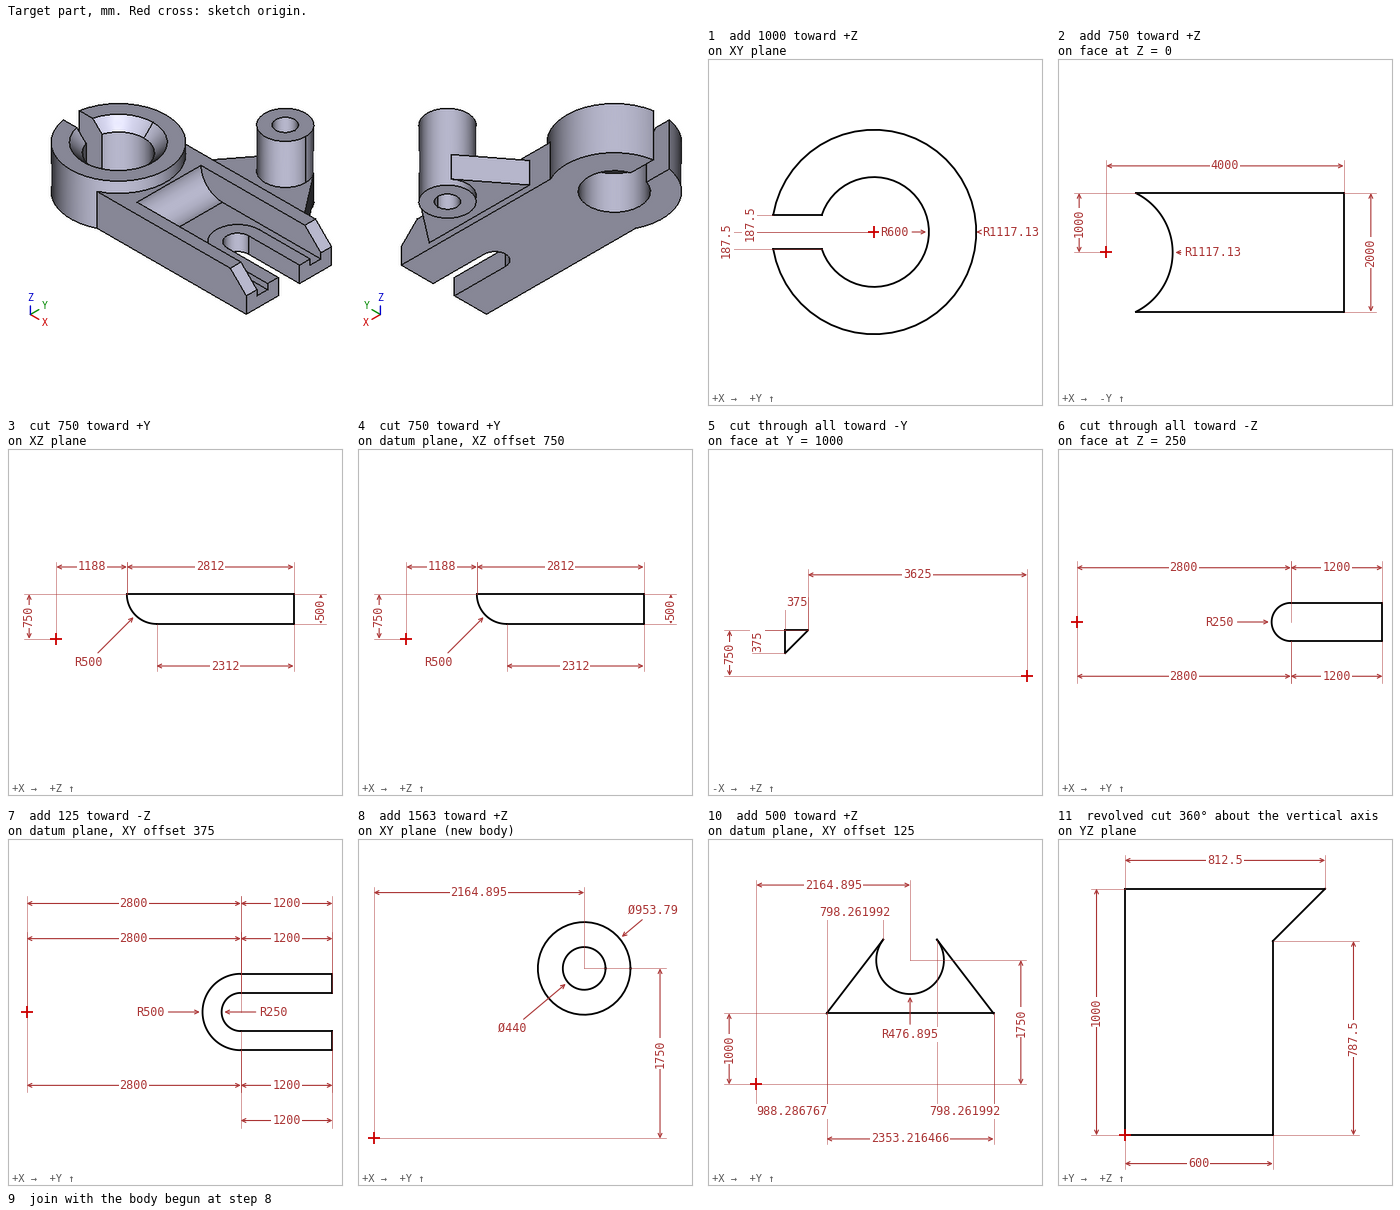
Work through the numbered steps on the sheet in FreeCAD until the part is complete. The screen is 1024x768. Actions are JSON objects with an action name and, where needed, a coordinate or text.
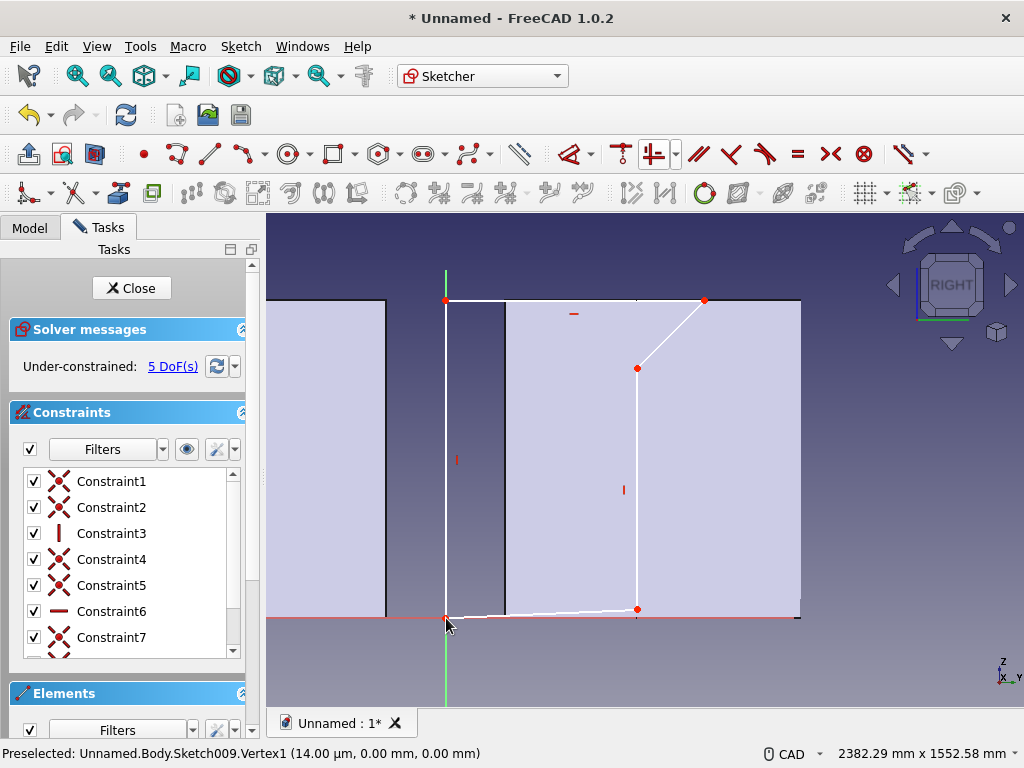
{"action": "left_click", "coordinate": [503, 616]}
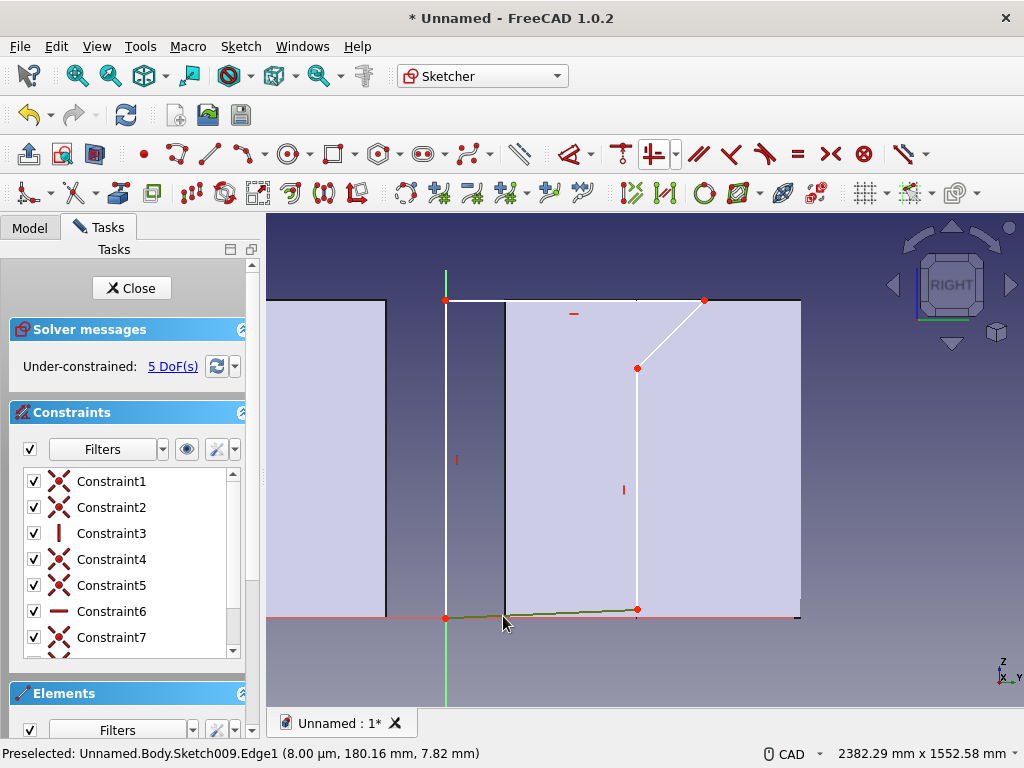
{"action": "left_click", "coordinate": [676, 154]}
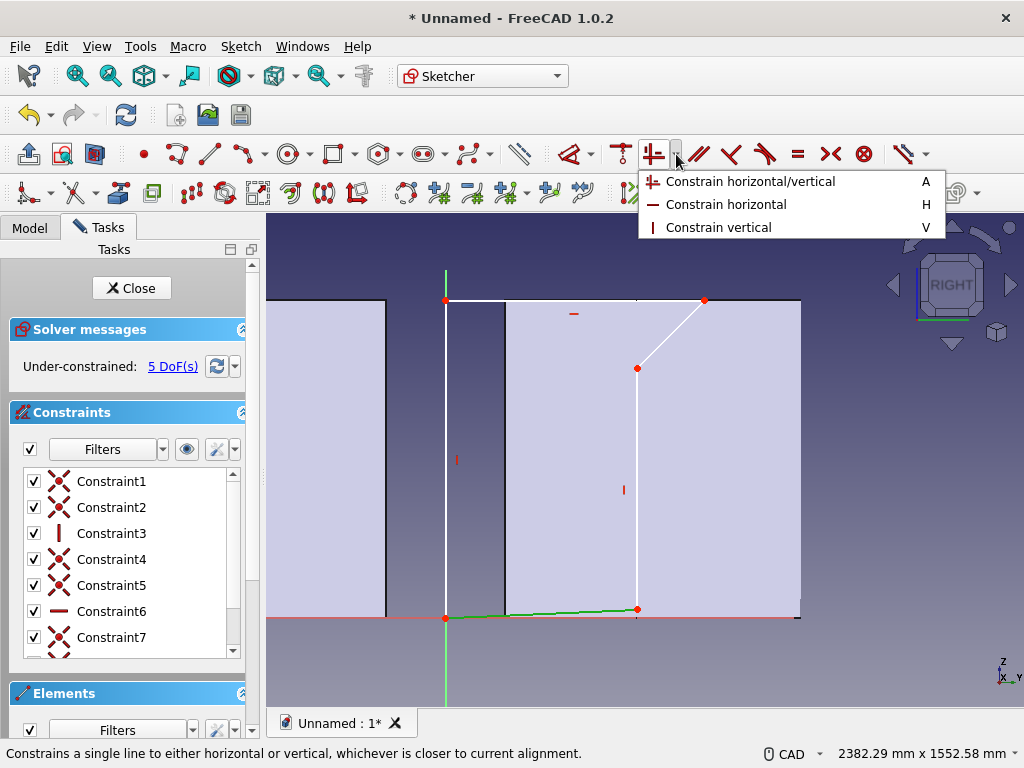
{"action": "left_click", "coordinate": [792, 204]}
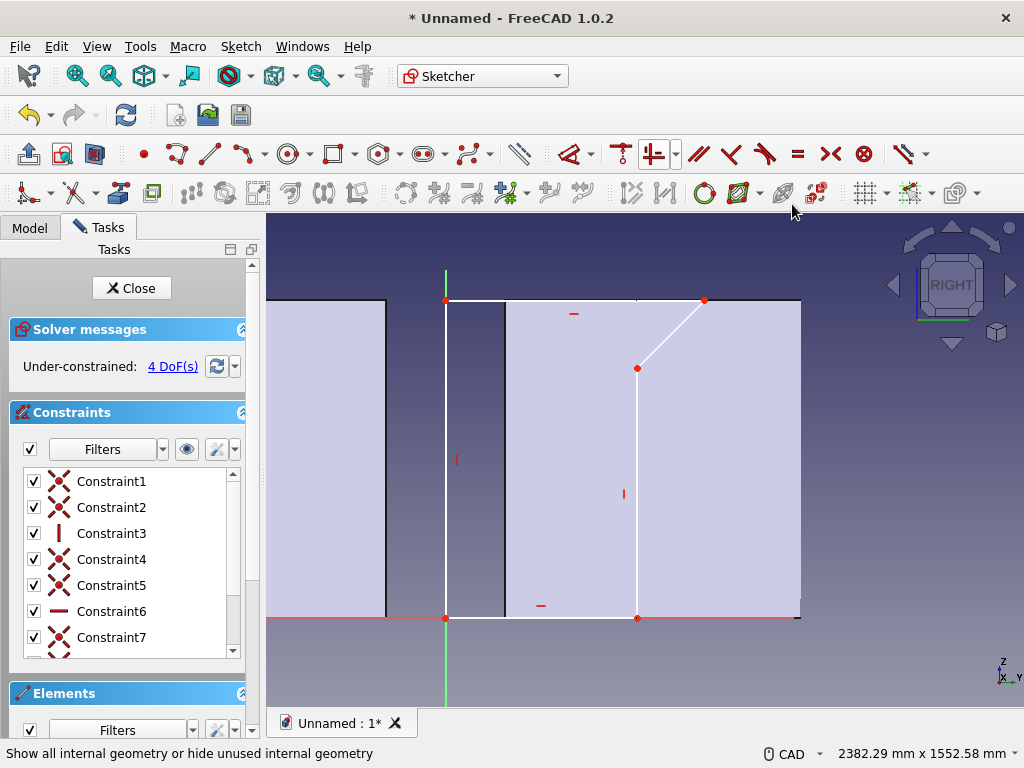
{"action": "key", "text": "d"}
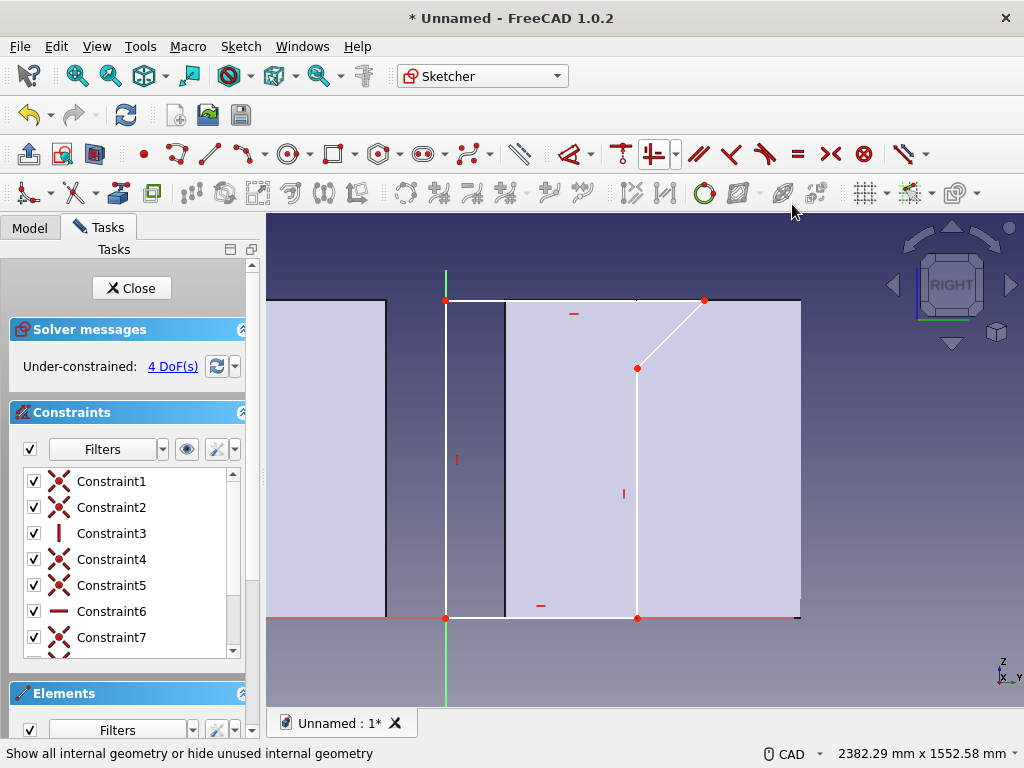
{"action": "left_click", "coordinate": [503, 618]}
{"action": "left_click", "coordinate": [541, 652]}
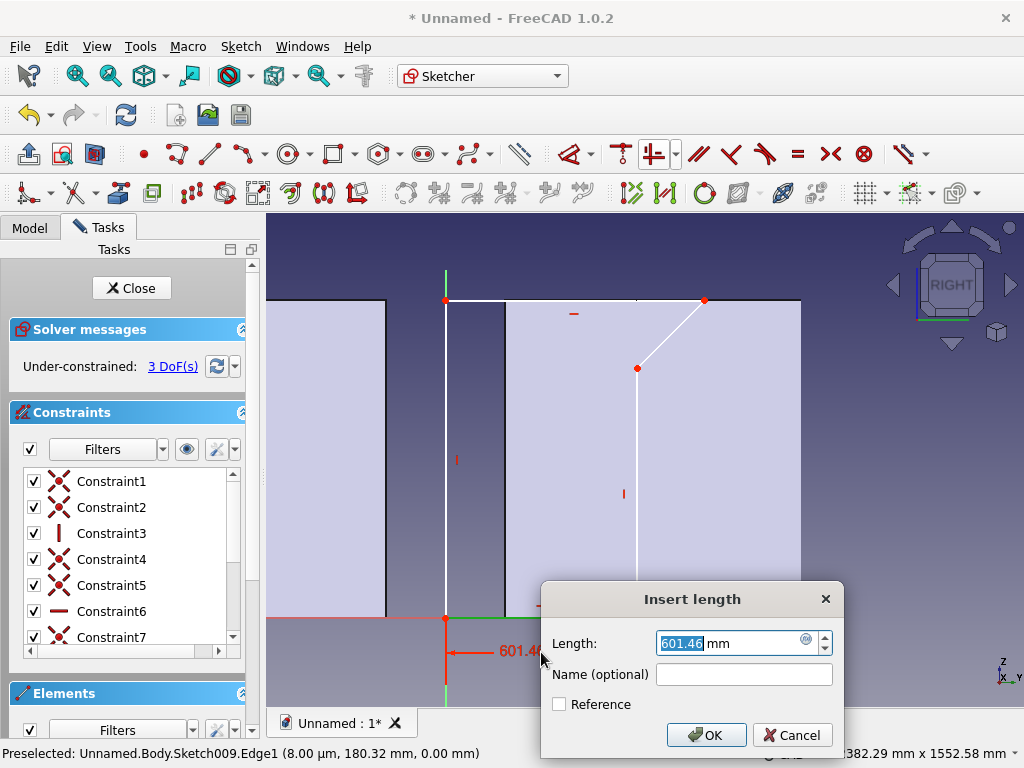
{"action": "type", "text": "600"}
{"action": "key", "text": "Return"}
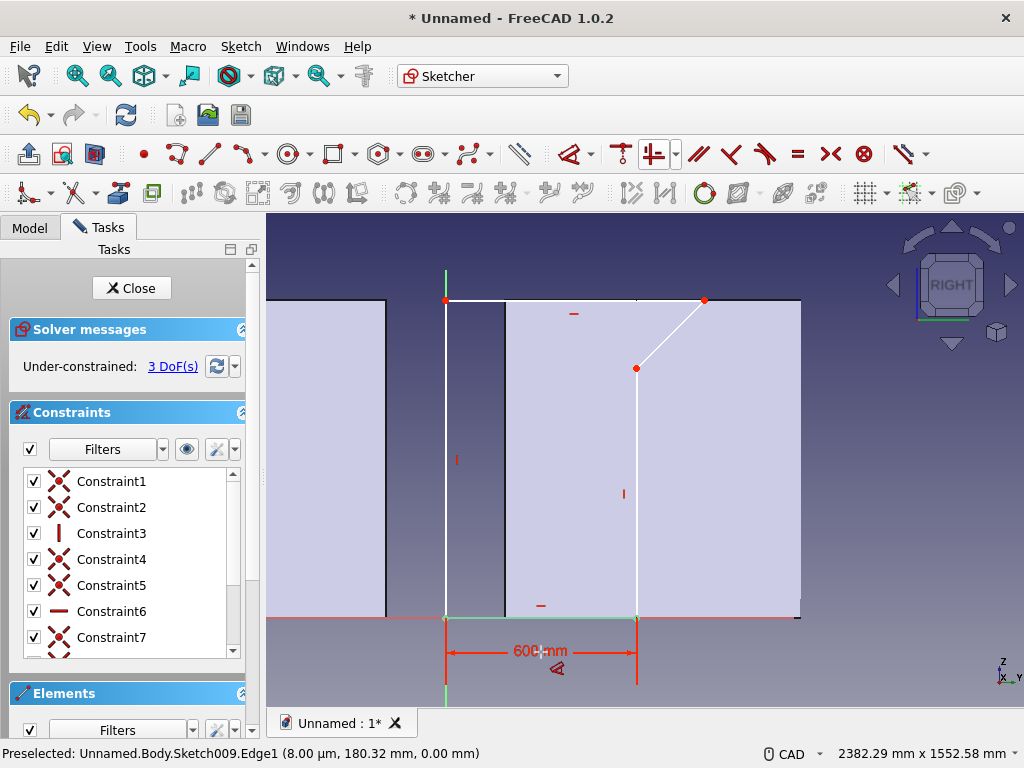
{"action": "left_click", "coordinate": [446, 396]}
{"action": "left_click", "coordinate": [412, 460]}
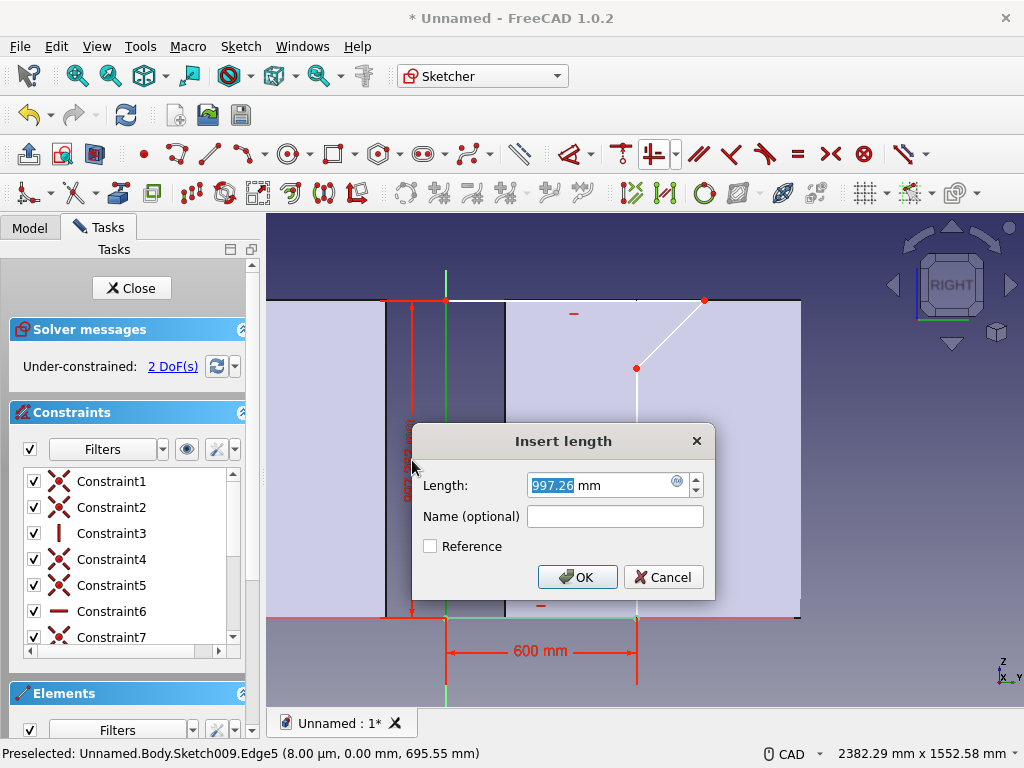
{"action": "type", "text": "1000"}
{"action": "key", "text": "Return"}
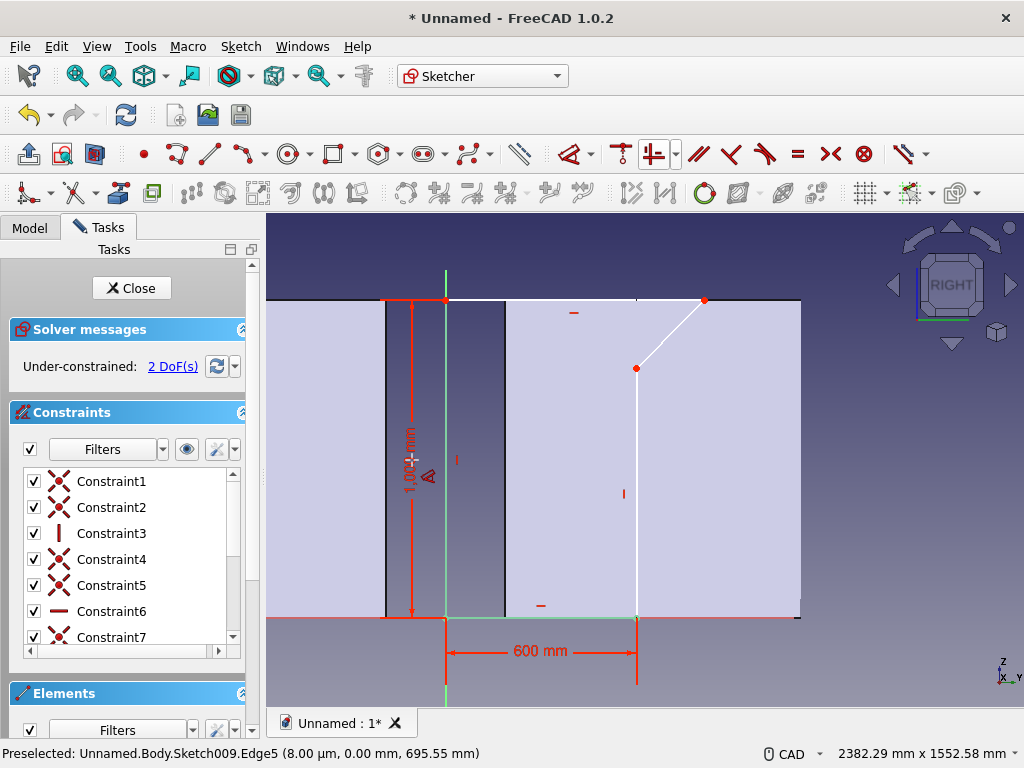
{"action": "left_click", "coordinate": [637, 544]}
{"action": "left_click", "coordinate": [671, 494]}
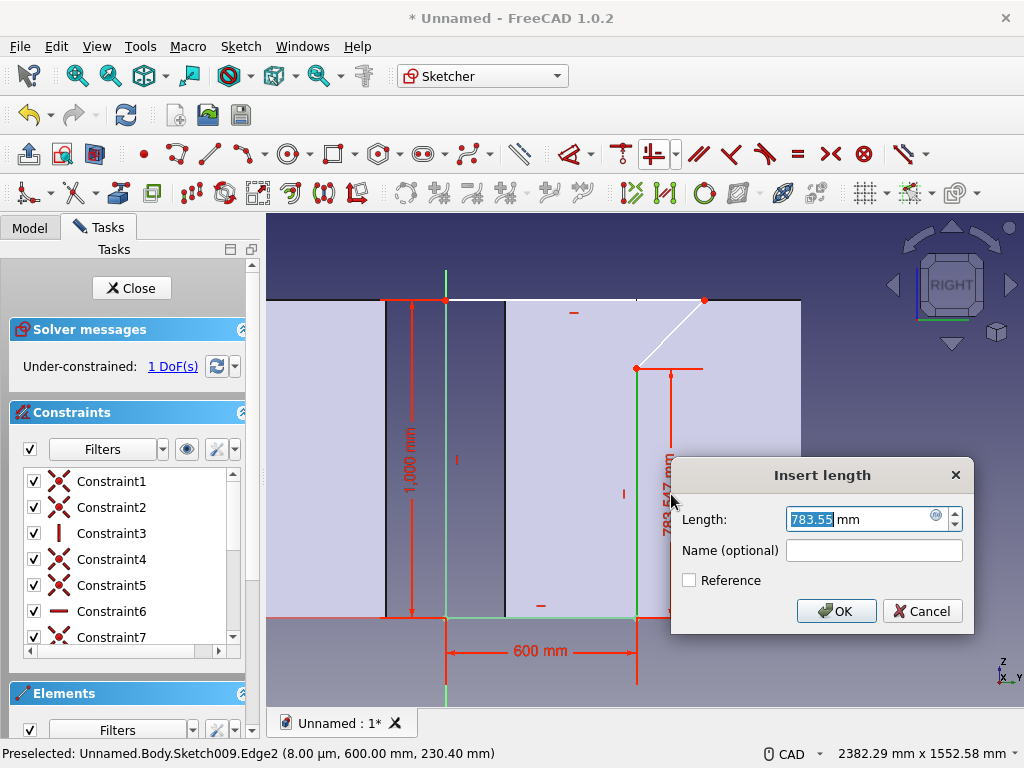
{"action": "type", "text": "787.5"}
{"action": "key", "text": "Return"}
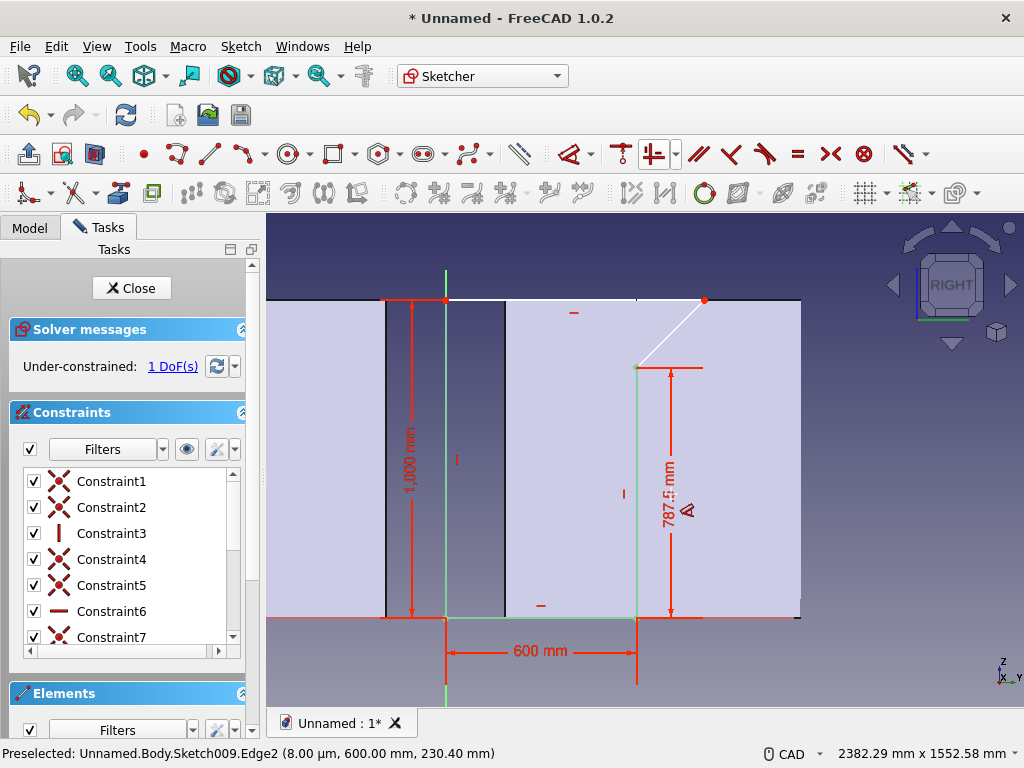
{"action": "left_click", "coordinate": [626, 300]}
{"action": "left_click", "coordinate": [575, 266]}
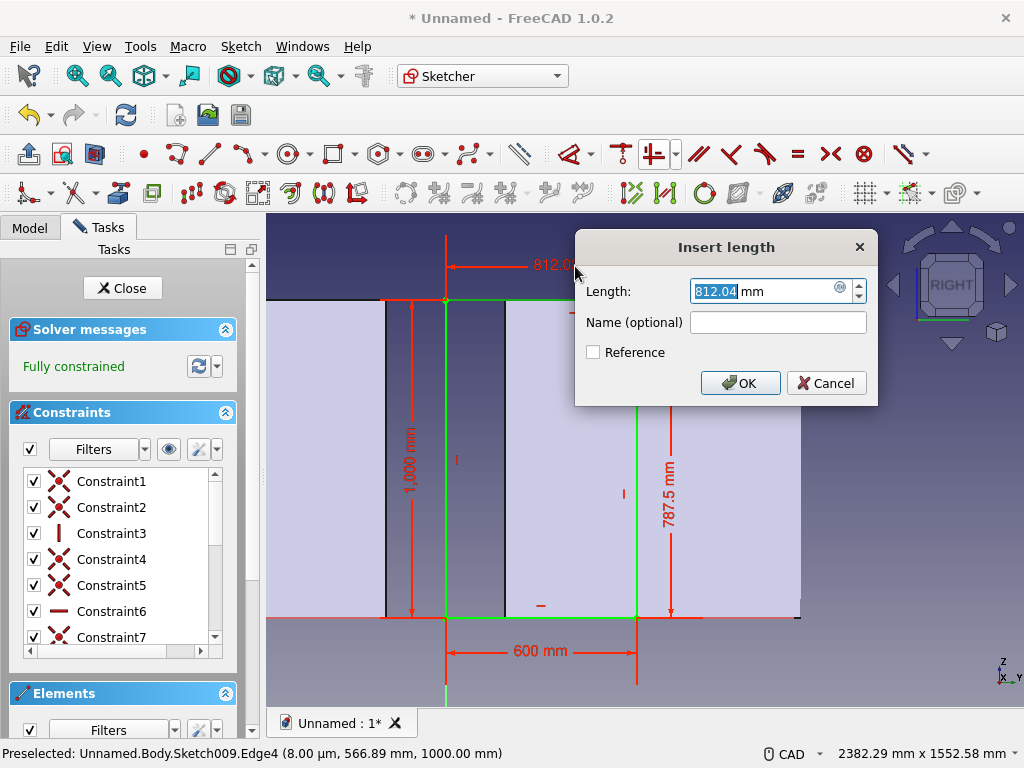
{"action": "type", "text": "812.5"}
{"action": "key", "text": "Return"}
{"action": "key", "text": "Escape"}